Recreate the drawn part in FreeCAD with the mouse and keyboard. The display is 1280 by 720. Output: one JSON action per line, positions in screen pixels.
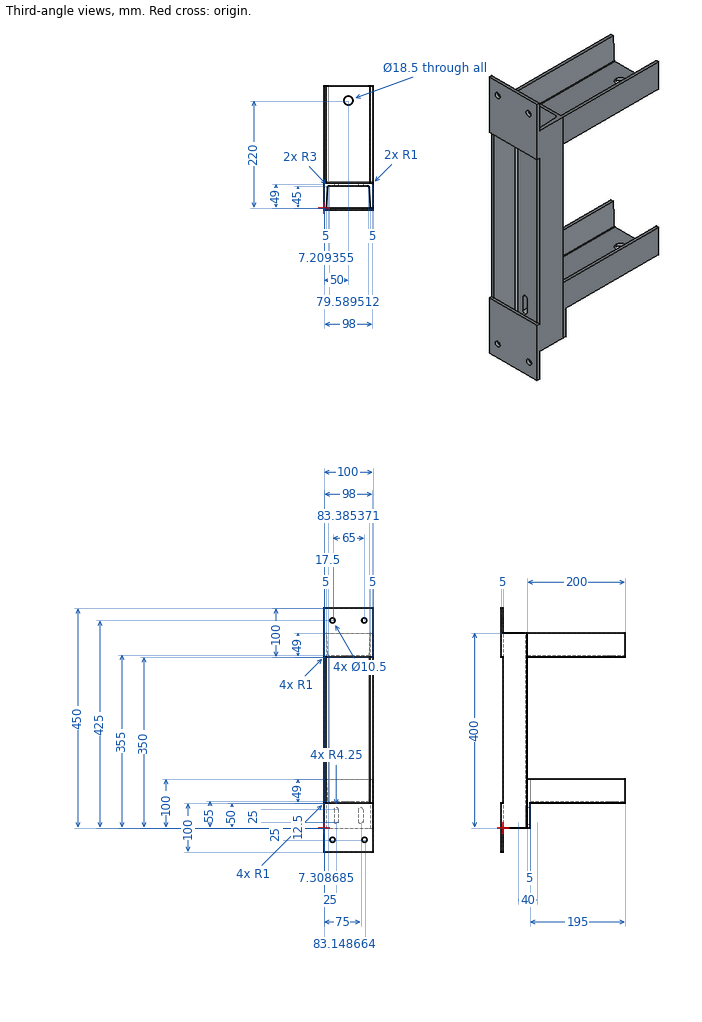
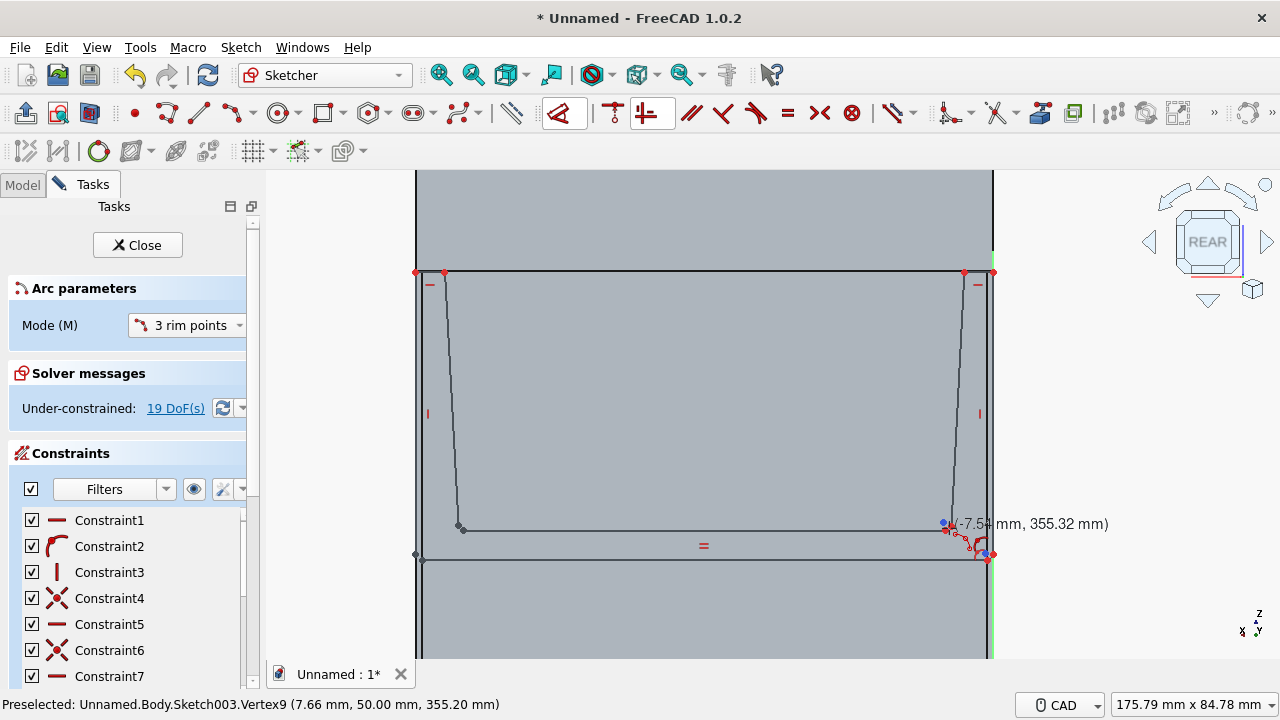
{"action": "scroll", "coordinate": [464, 531], "scroll_direction": "up", "scroll_amount": 4}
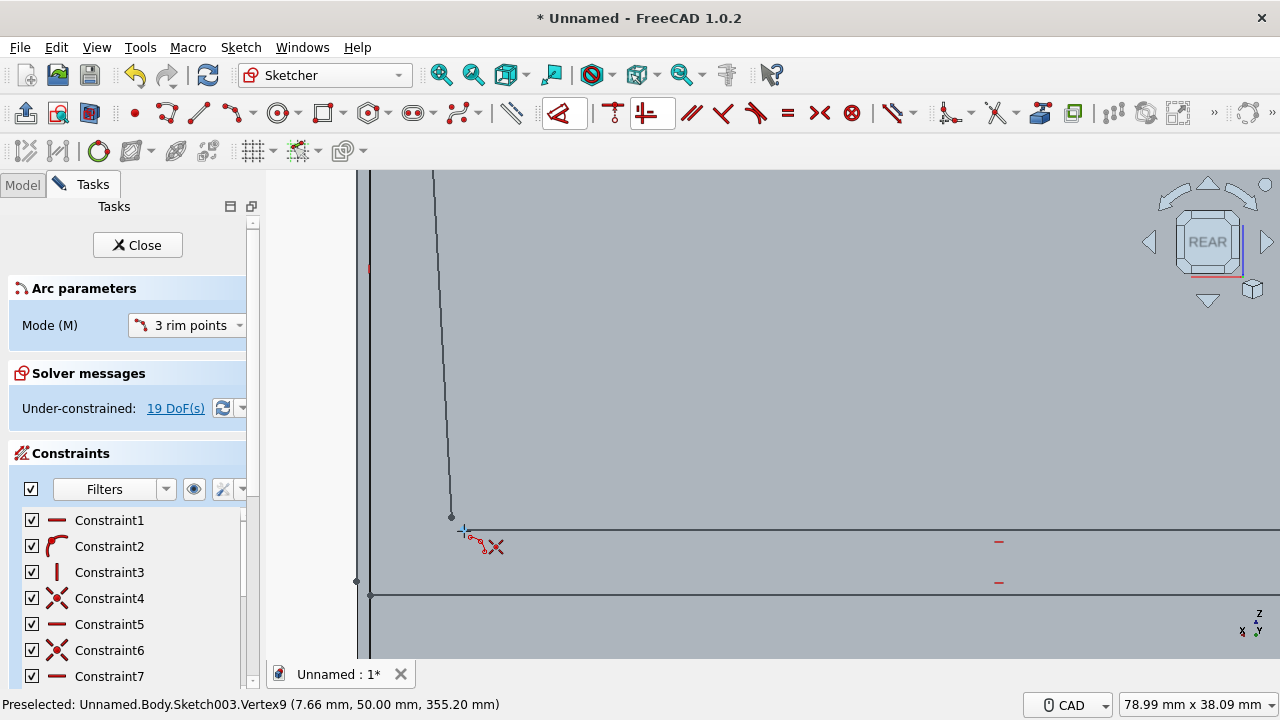
{"action": "left_click", "coordinate": [464, 530]}
{"action": "left_click", "coordinate": [452, 518]}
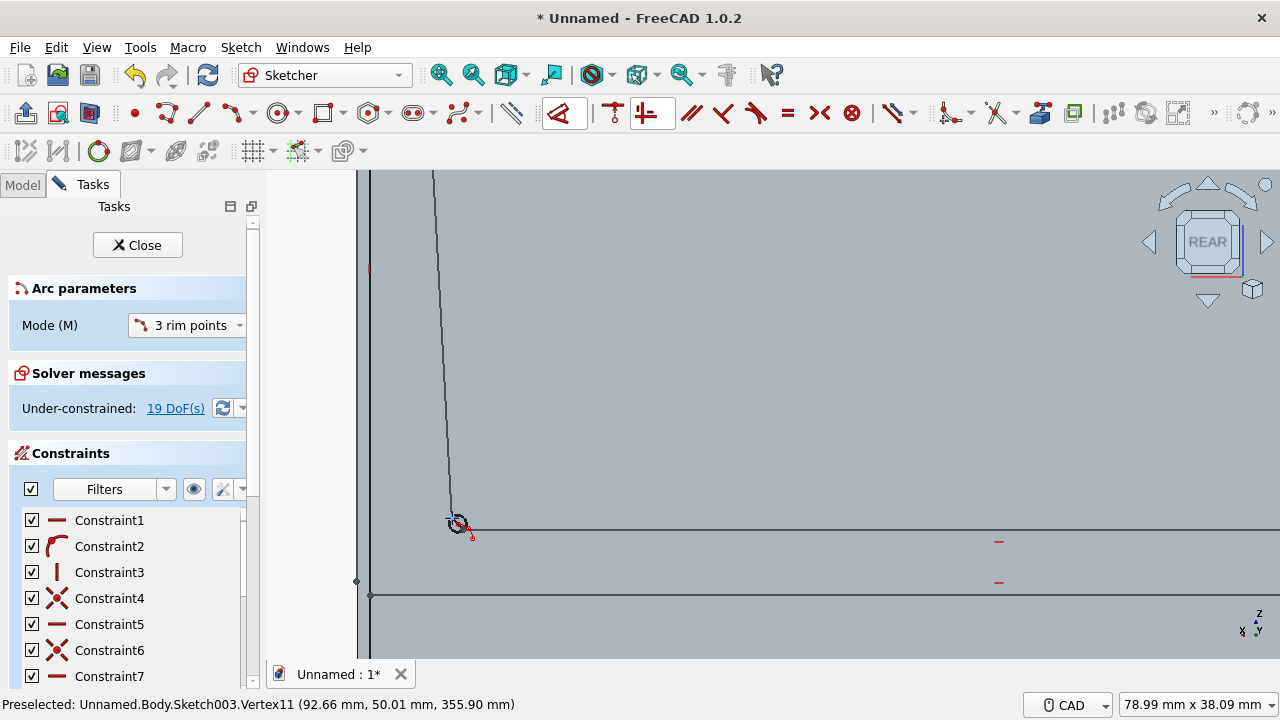
{"action": "scroll", "coordinate": [455, 526], "scroll_direction": "up", "scroll_amount": 8}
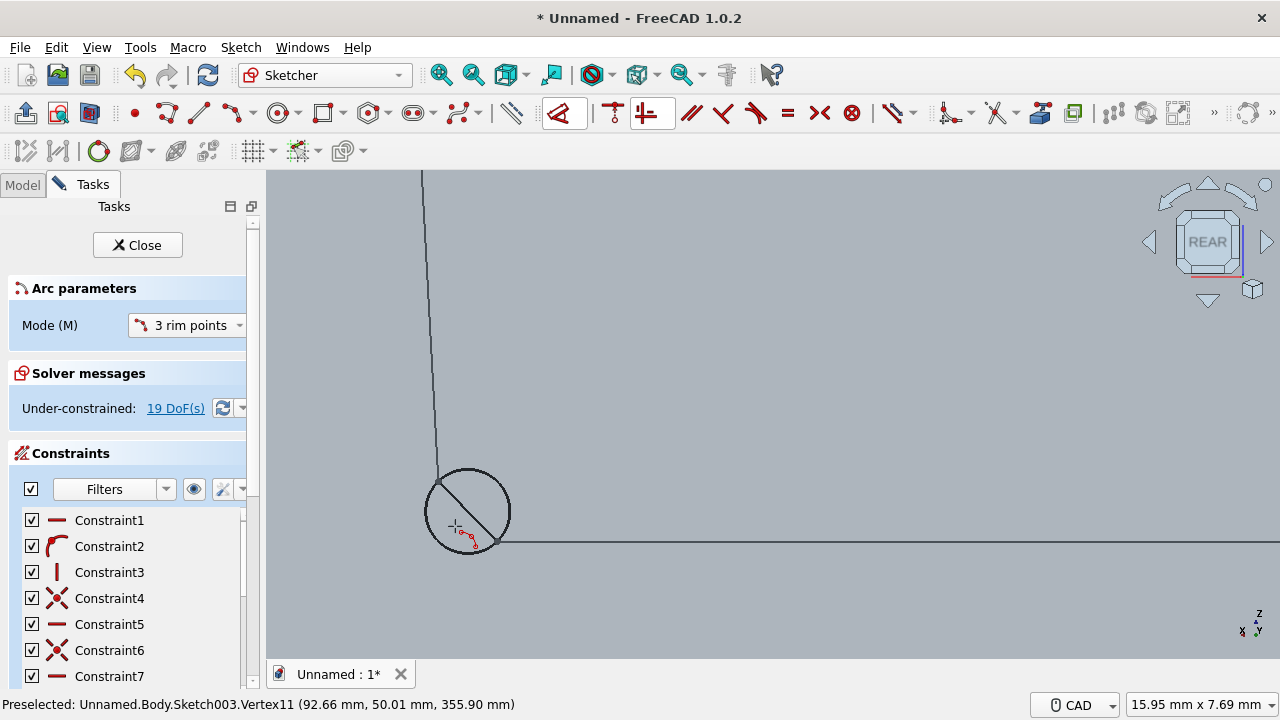
{"action": "left_click", "coordinate": [456, 521]}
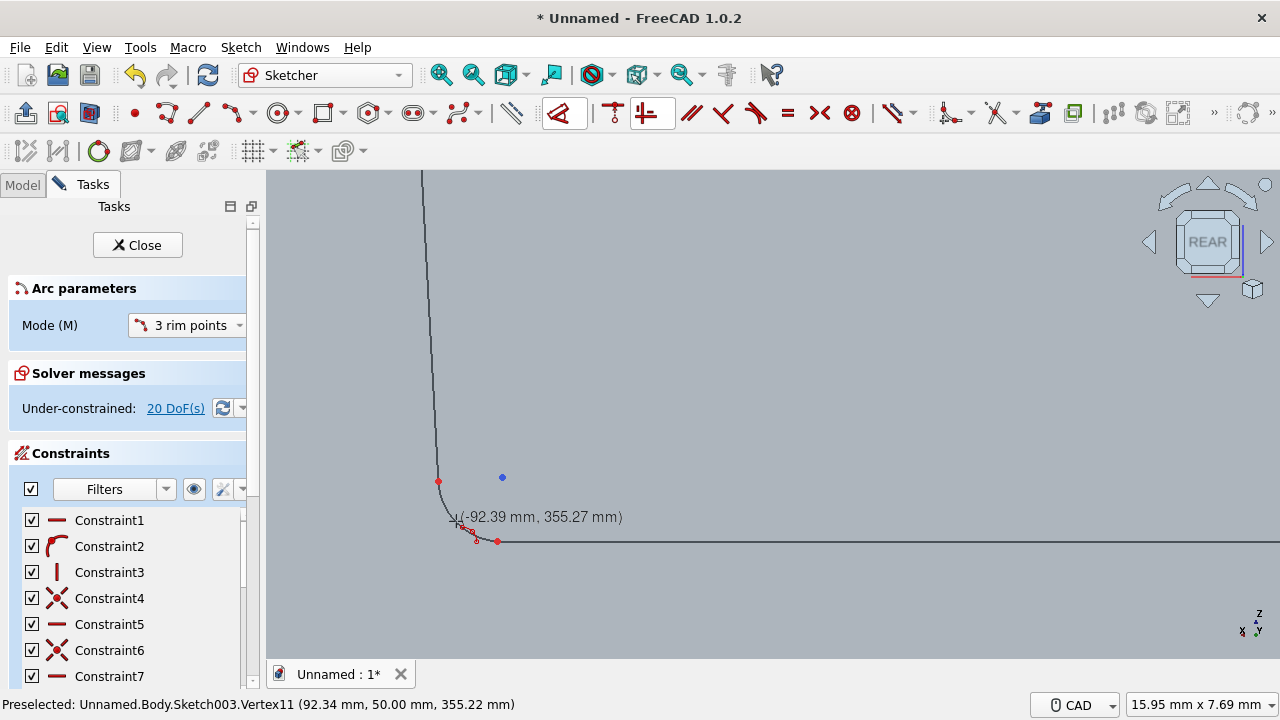
{"action": "scroll", "coordinate": [460, 529], "scroll_direction": "down", "scroll_amount": 12}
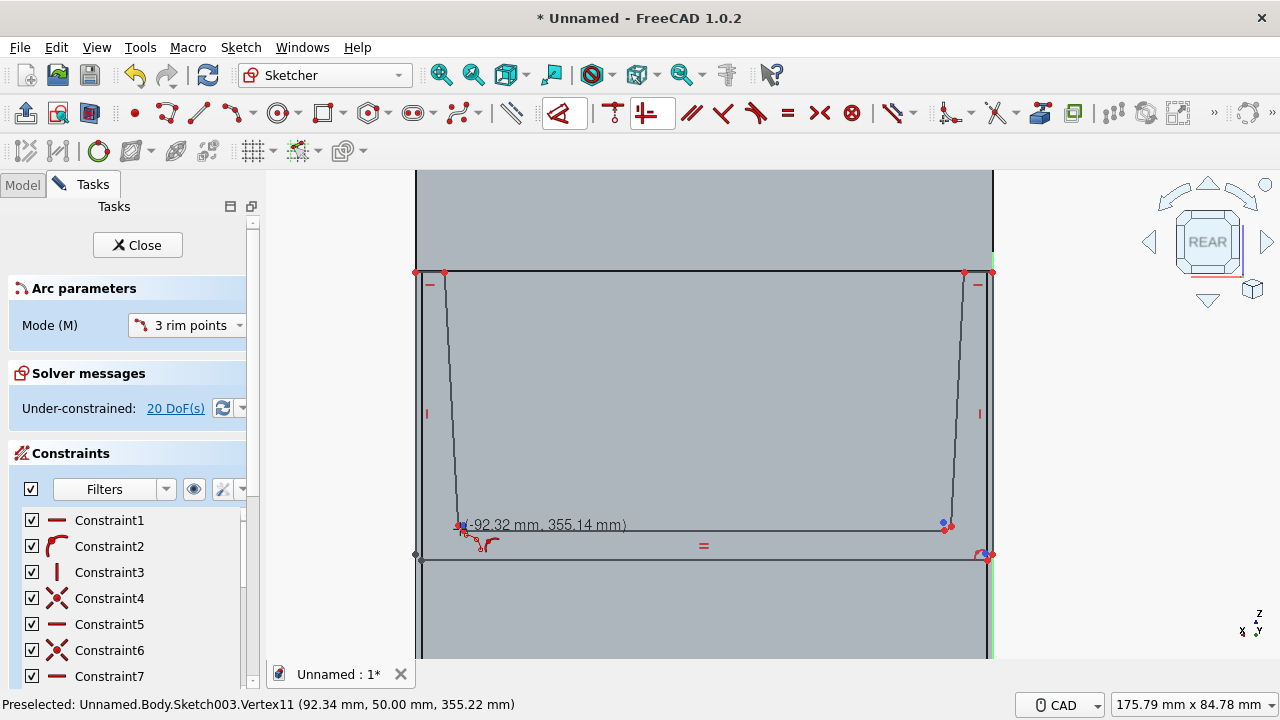
{"action": "scroll", "coordinate": [416, 554], "scroll_direction": "up", "scroll_amount": 4}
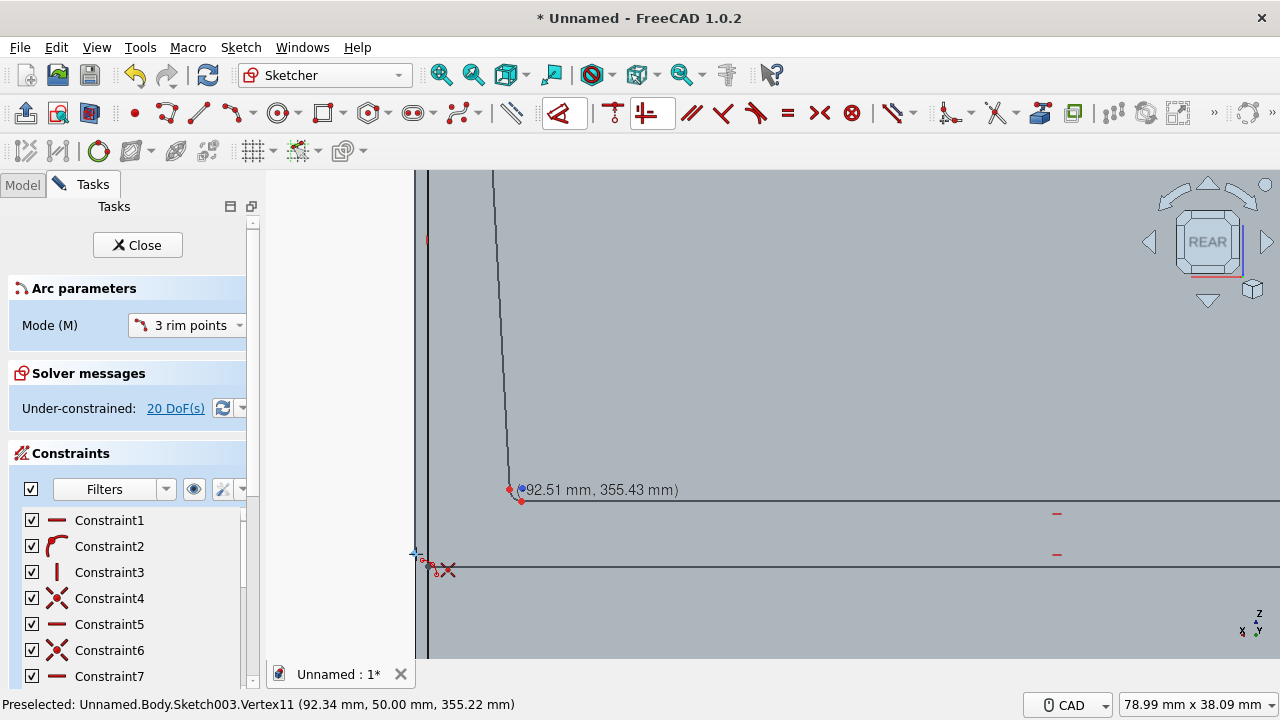
{"action": "left_click", "coordinate": [415, 554]}
{"action": "left_click", "coordinate": [428, 567]}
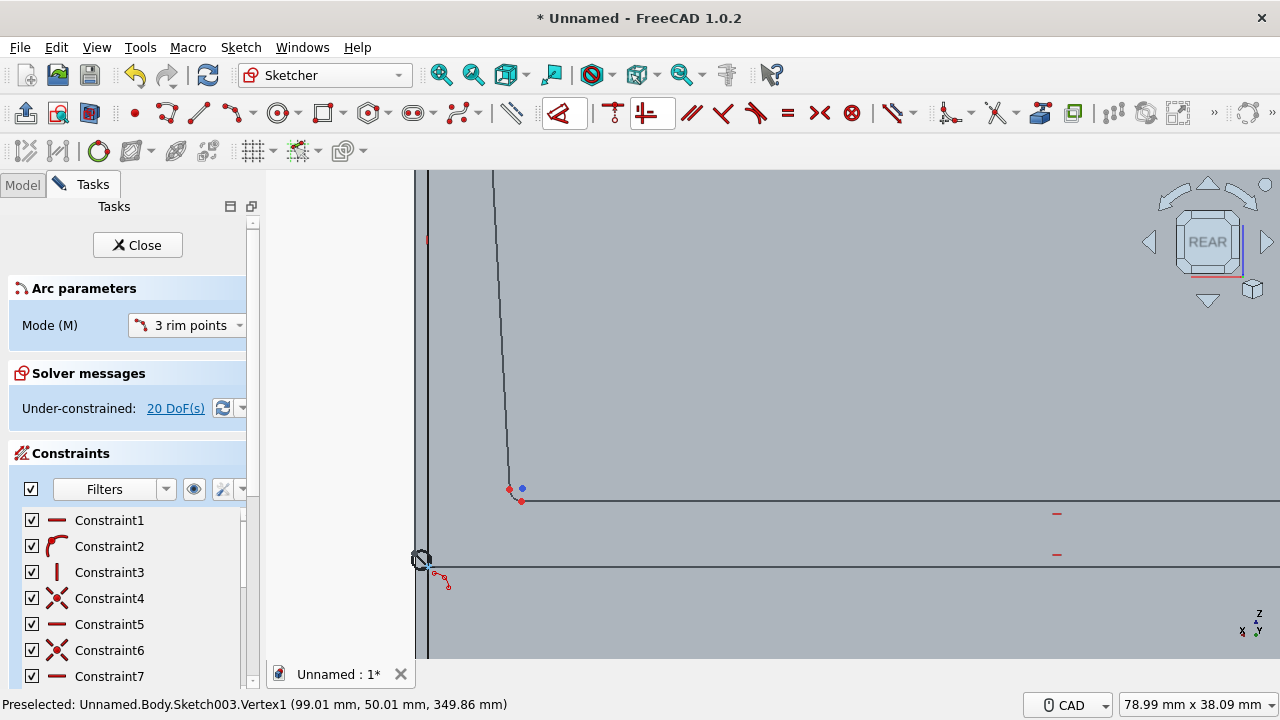
{"action": "scroll", "coordinate": [419, 561], "scroll_direction": "up", "scroll_amount": 8}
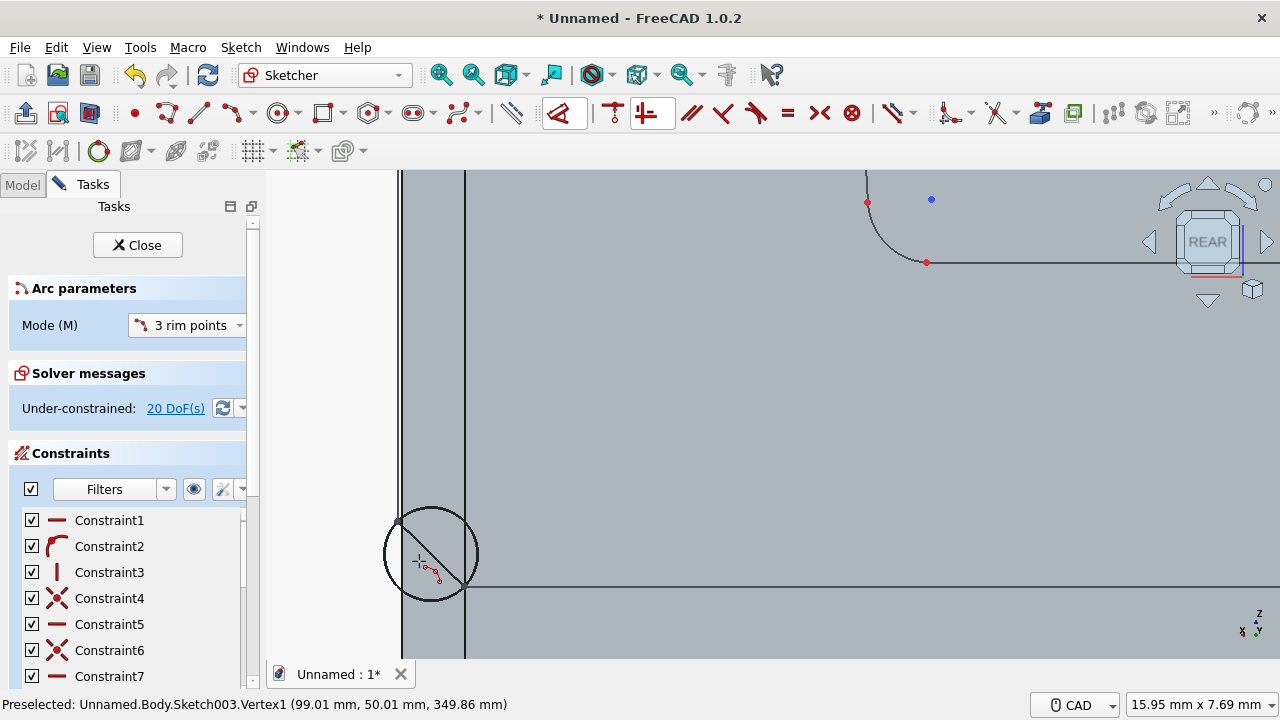
{"action": "left_click", "coordinate": [420, 559]}
{"action": "key", "text": "Escape"}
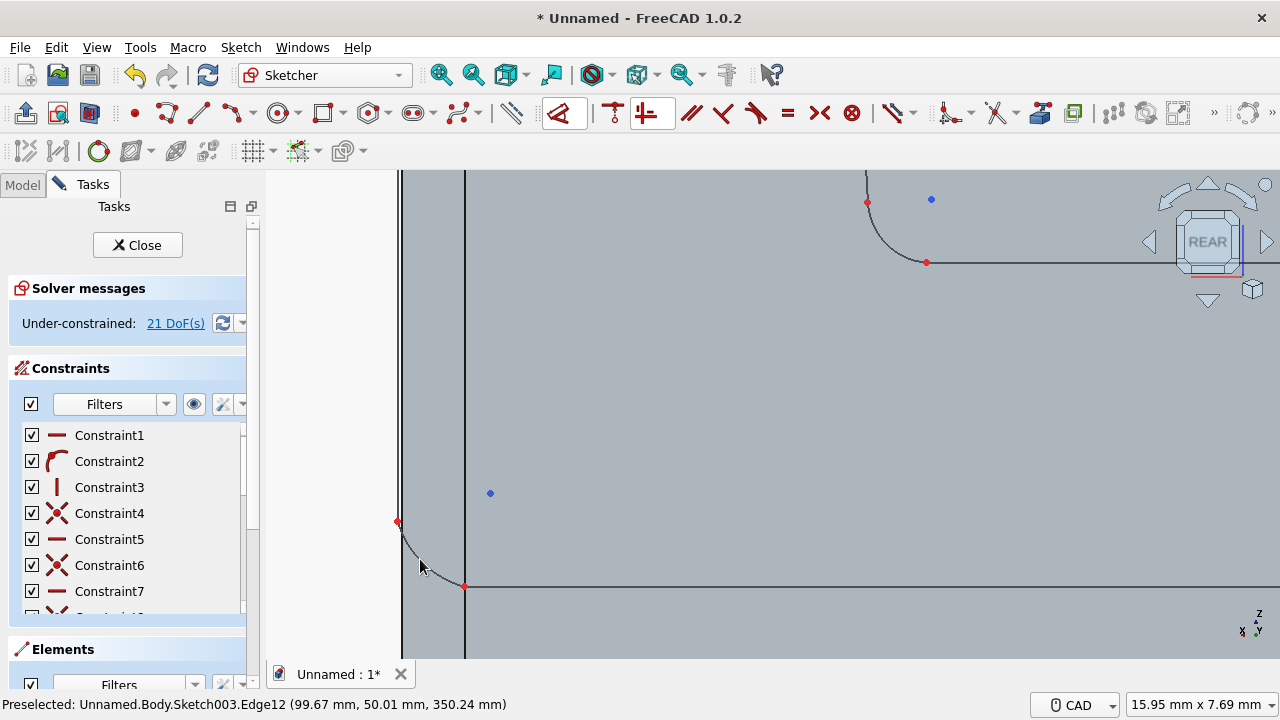
{"action": "scroll", "coordinate": [418, 557], "scroll_direction": "down", "scroll_amount": 12}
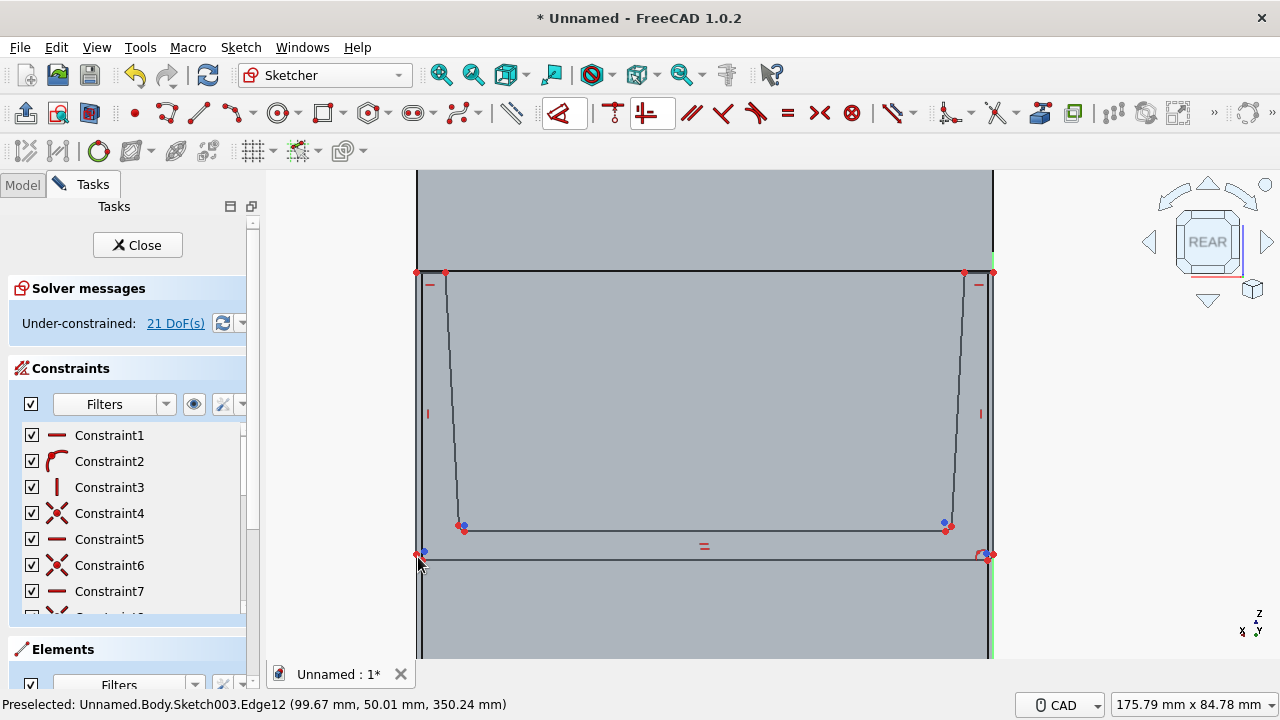
{"action": "left_click", "coordinate": [592, 560]}